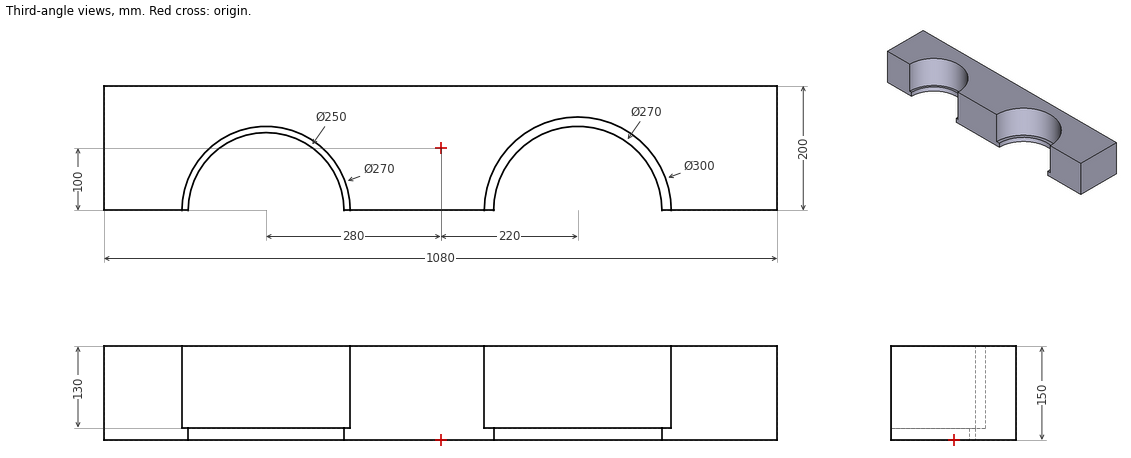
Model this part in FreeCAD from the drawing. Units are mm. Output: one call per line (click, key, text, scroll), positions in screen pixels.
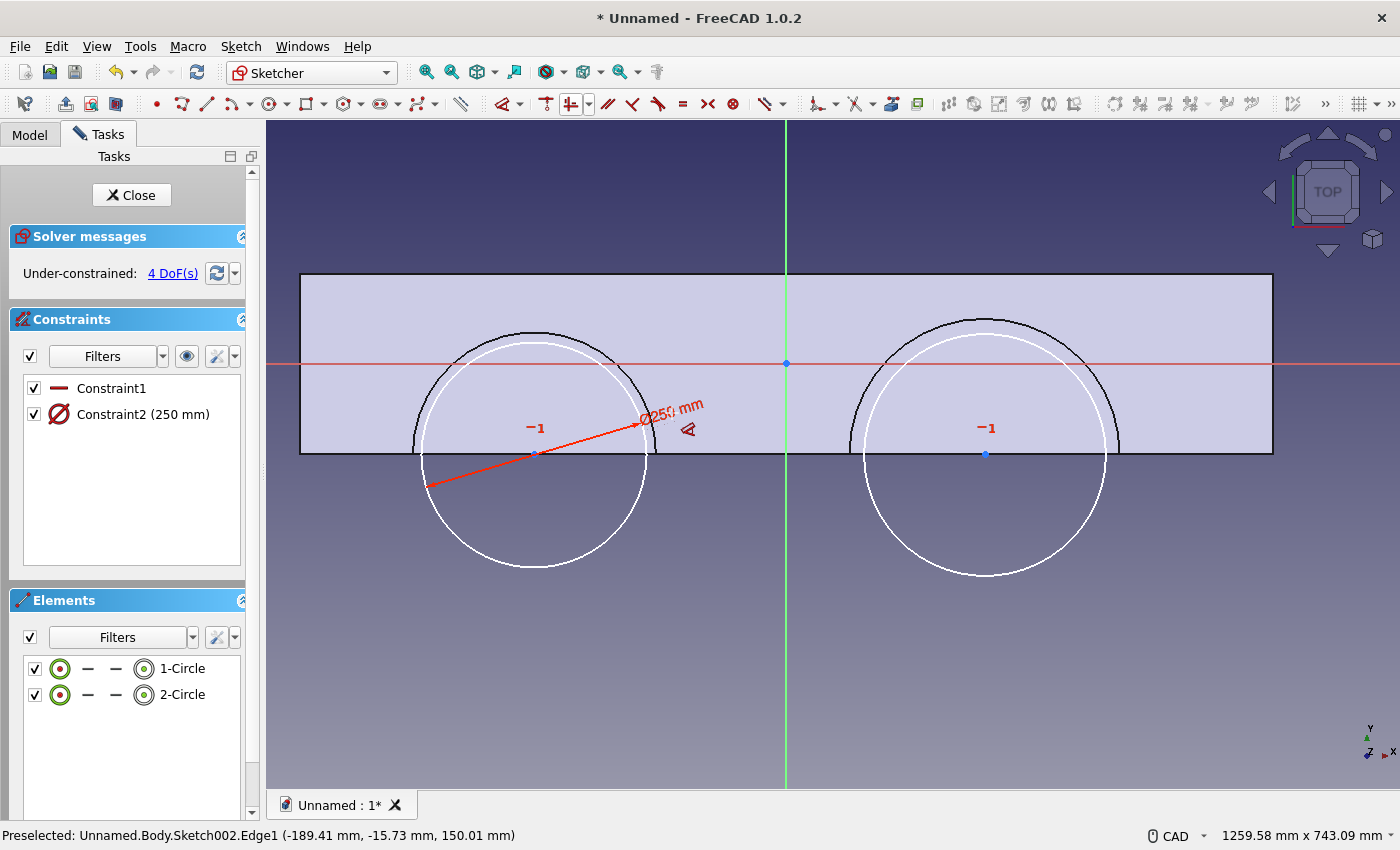
click(900, 541)
click(878, 564)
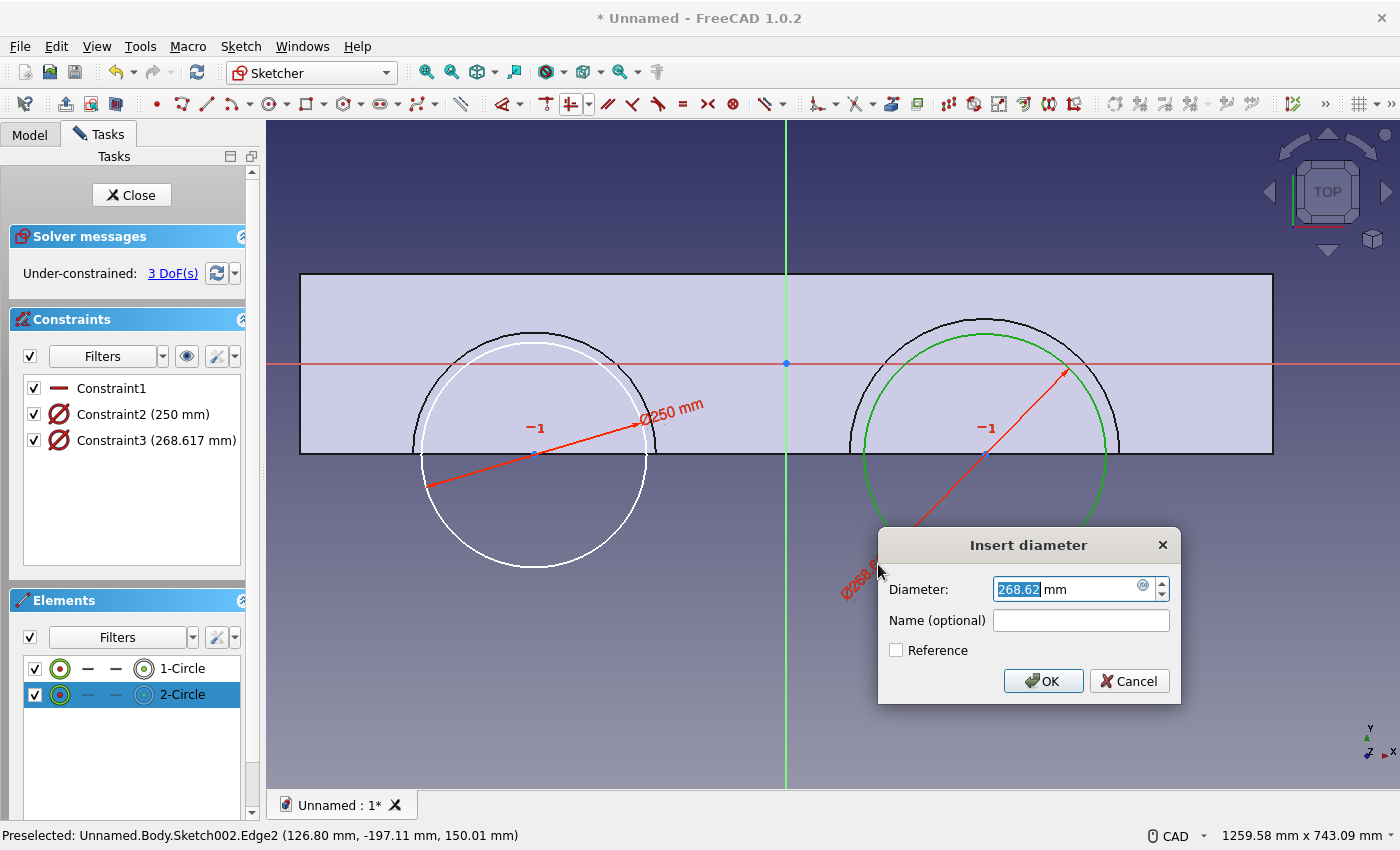
text(270)
key(Return)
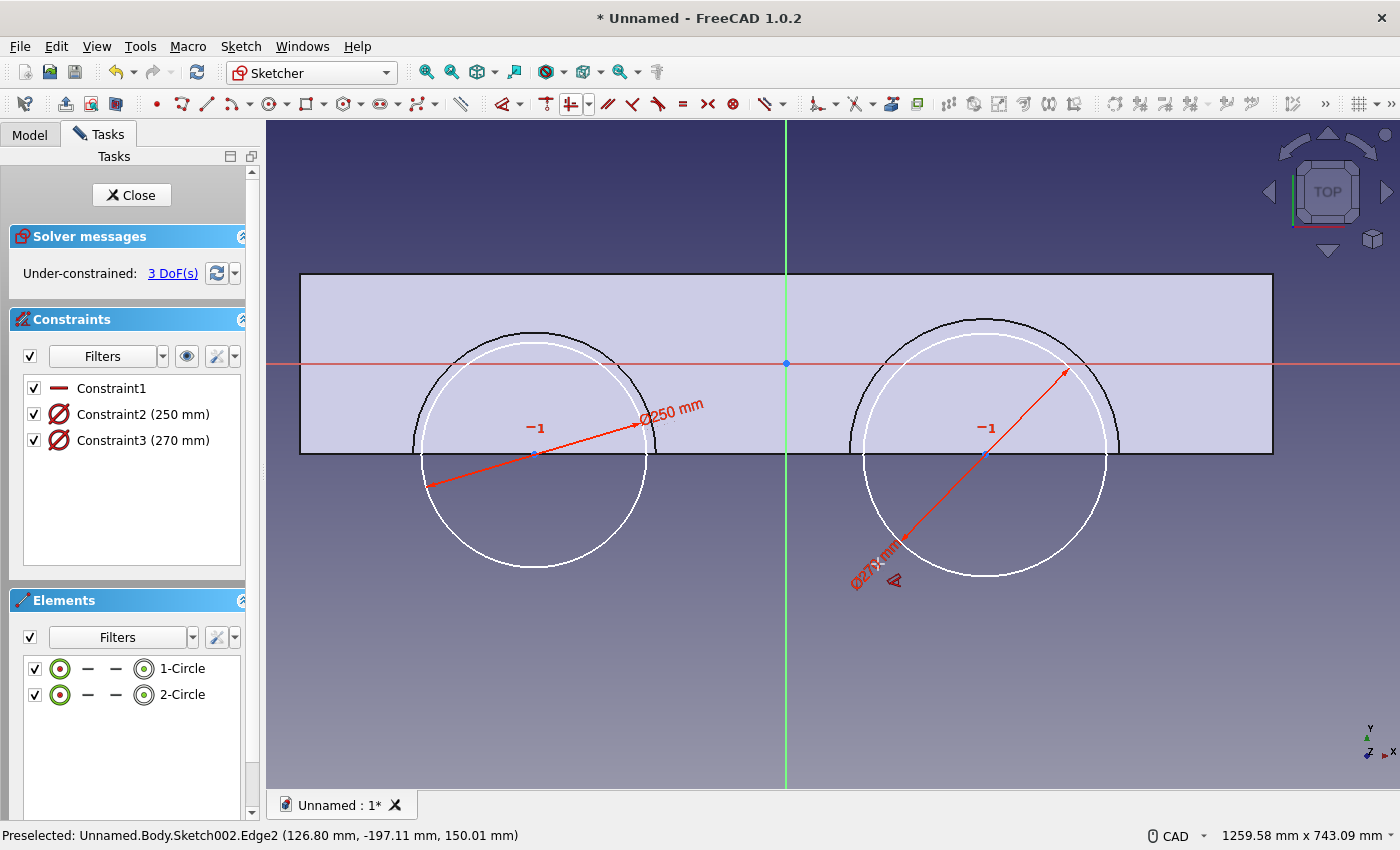
click(534, 455)
click(660, 330)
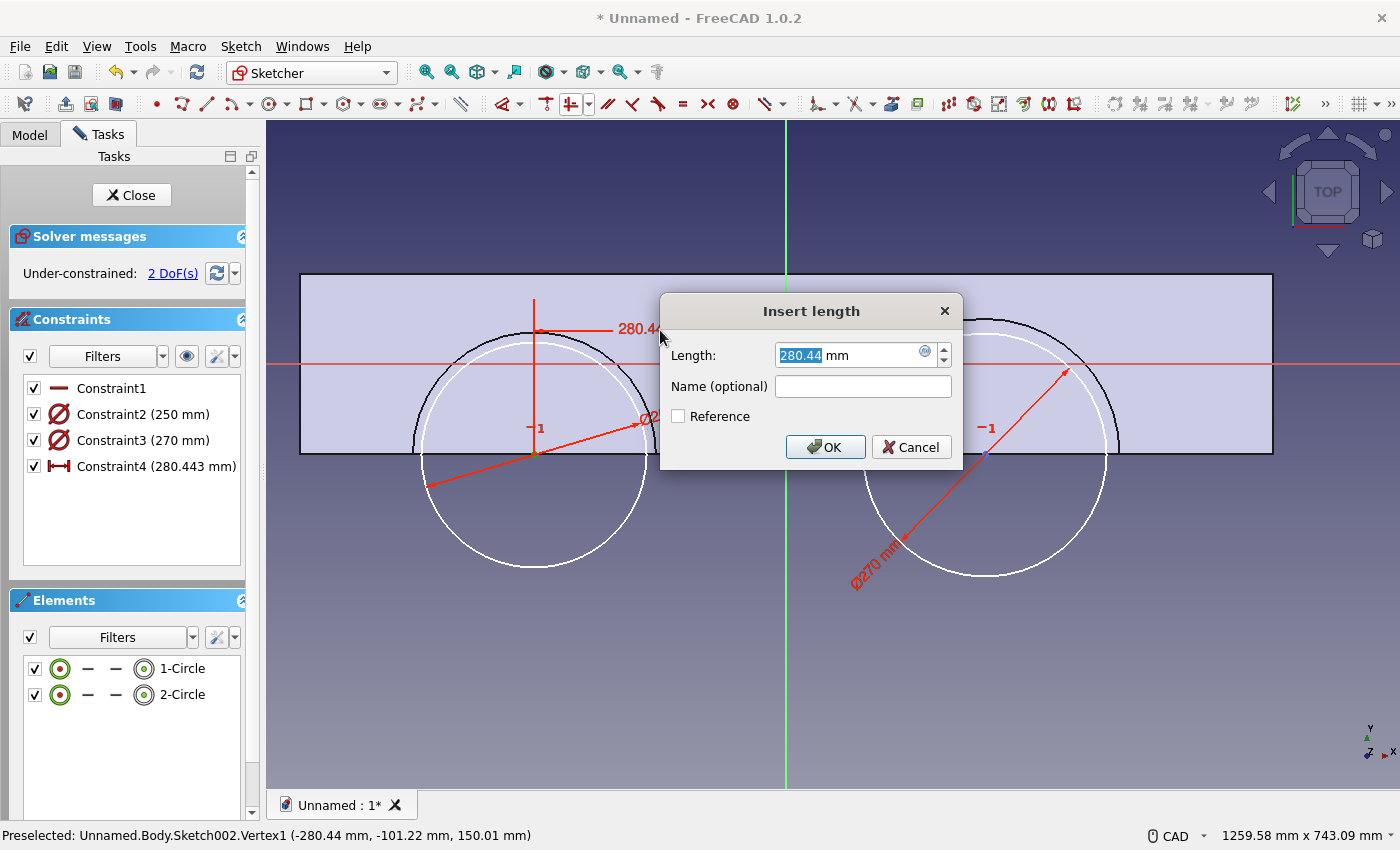
text(280)
key(Return)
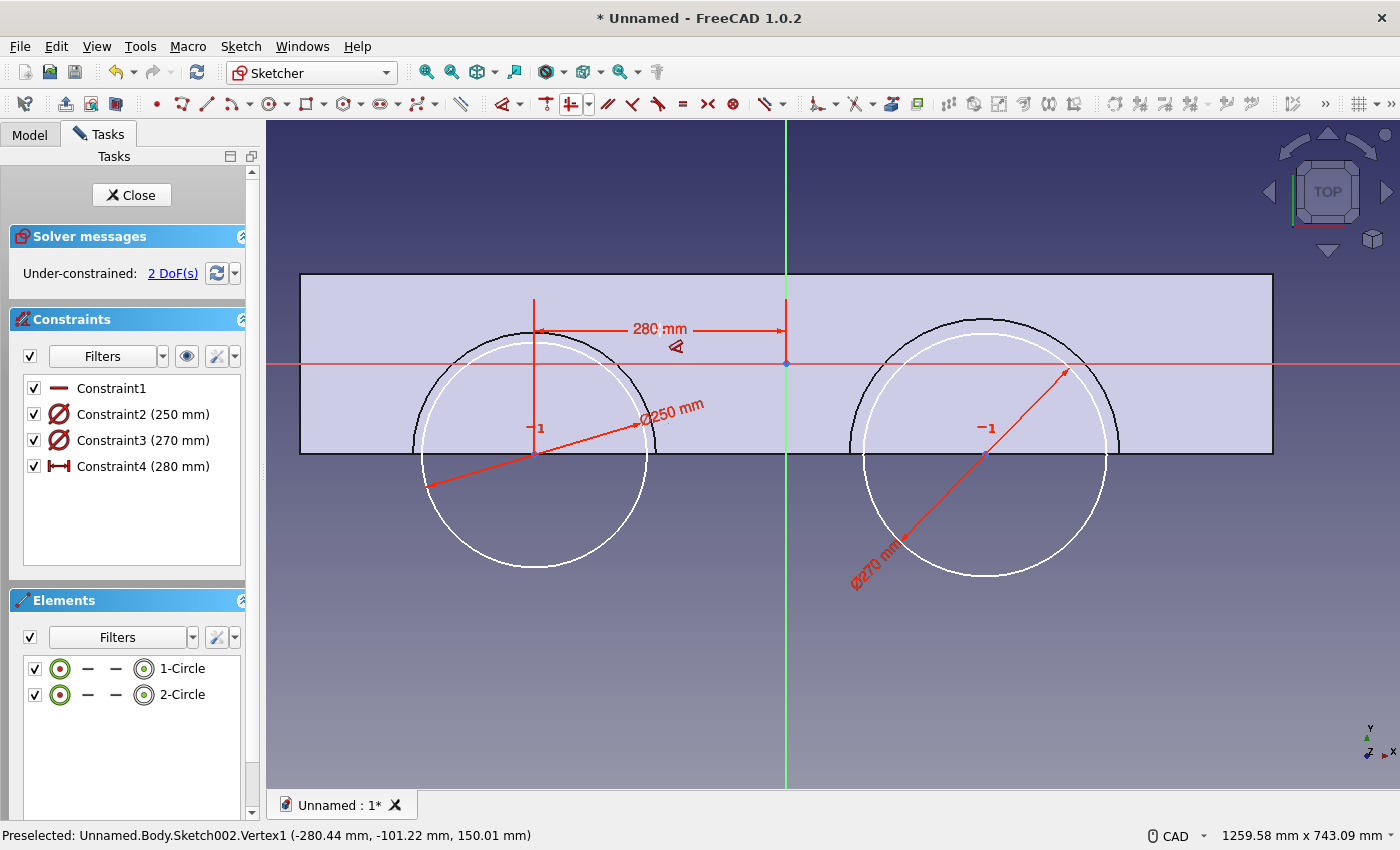
click(534, 455)
click(500, 409)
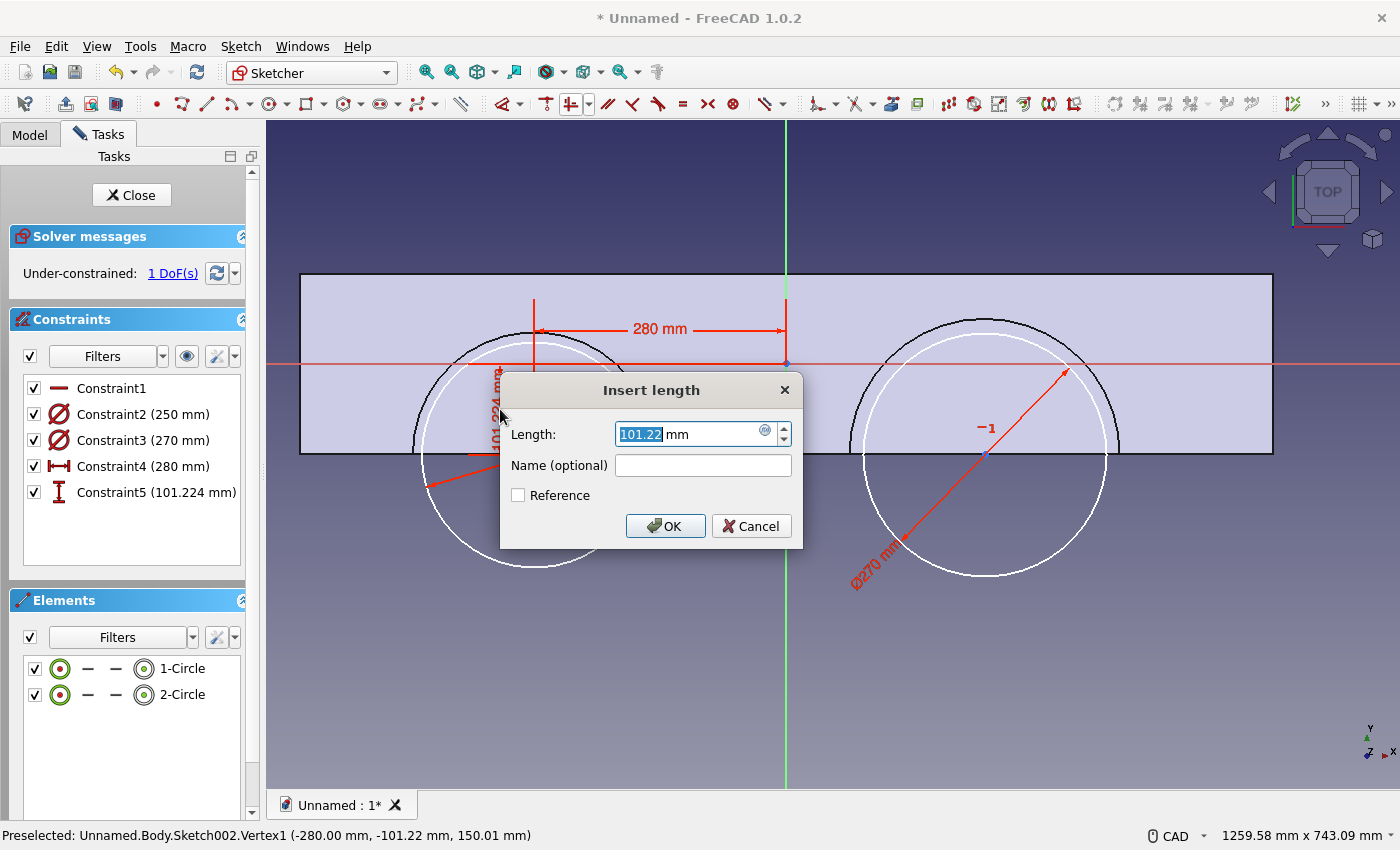
text(100)
key(Return)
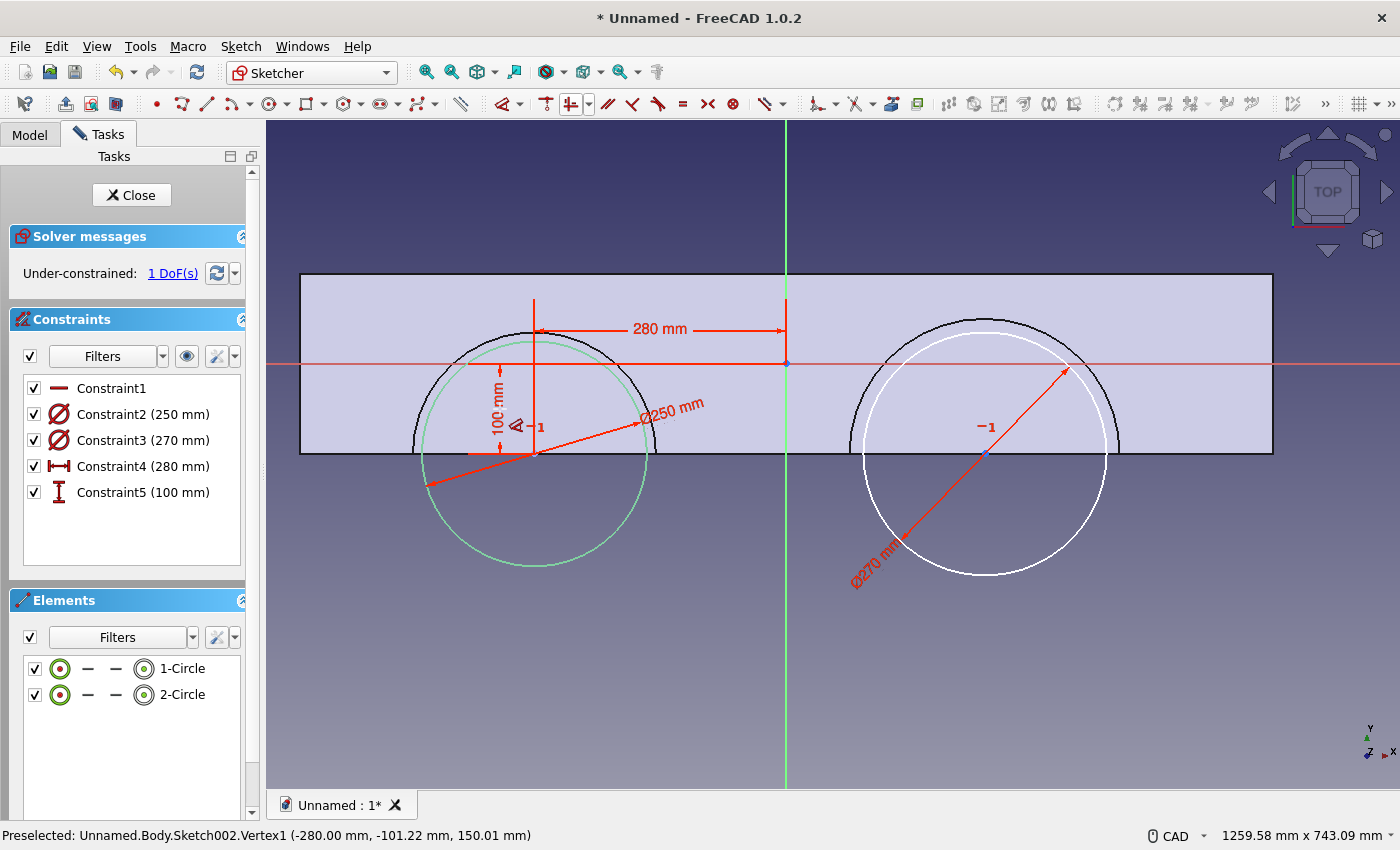
click(985, 454)
click(886, 330)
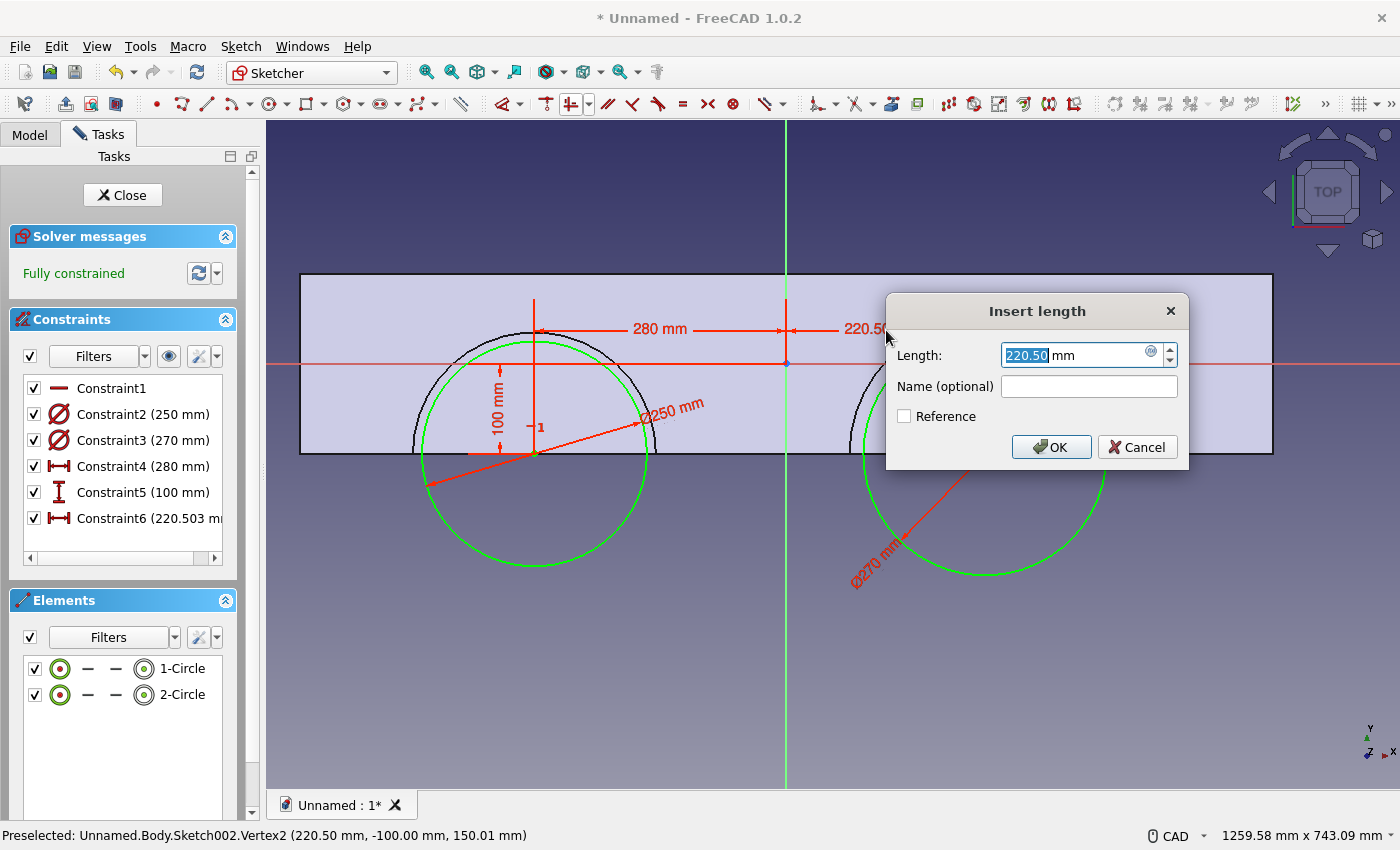
text(220)
key(Return)
key(Escape)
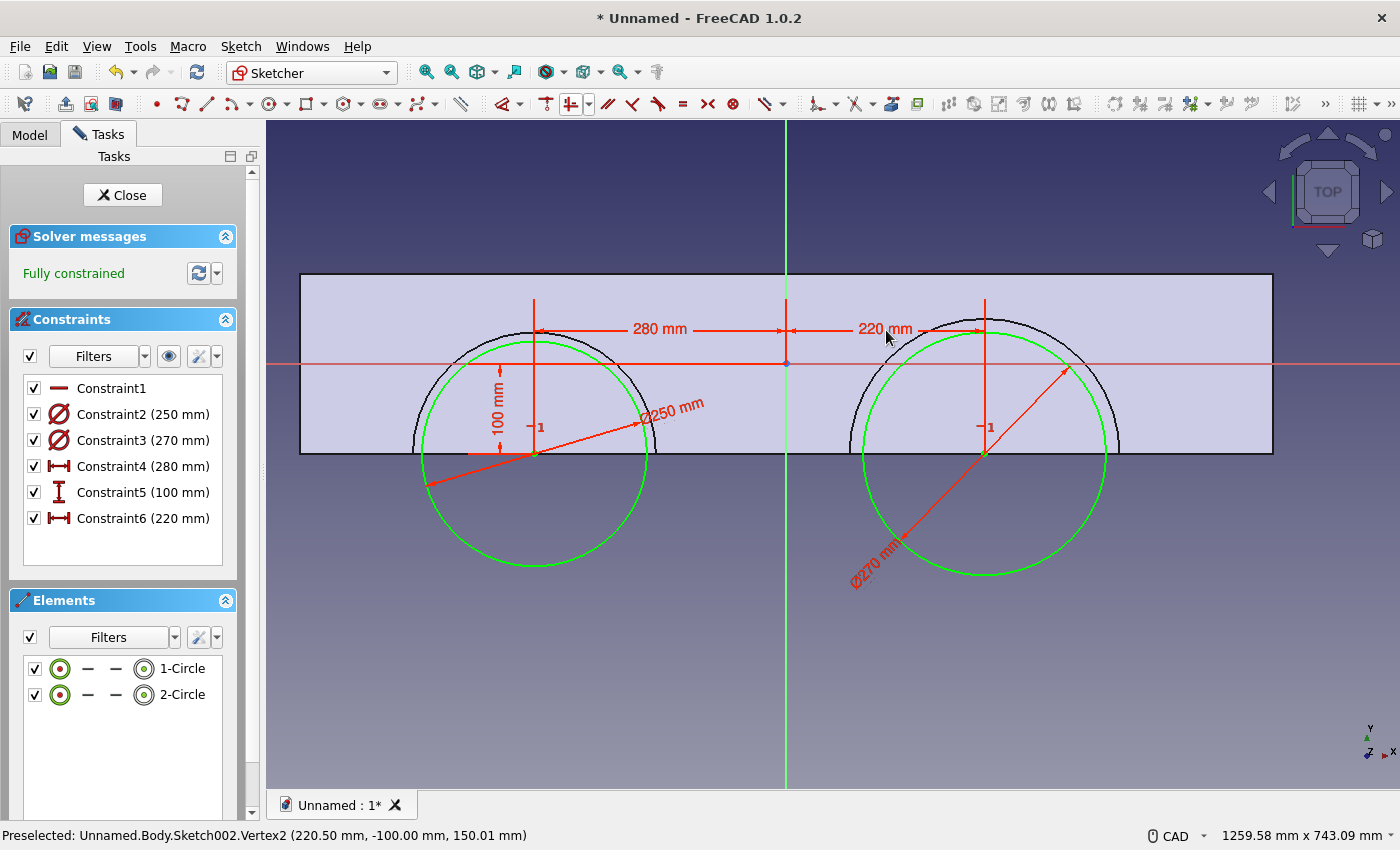
click(123, 195)